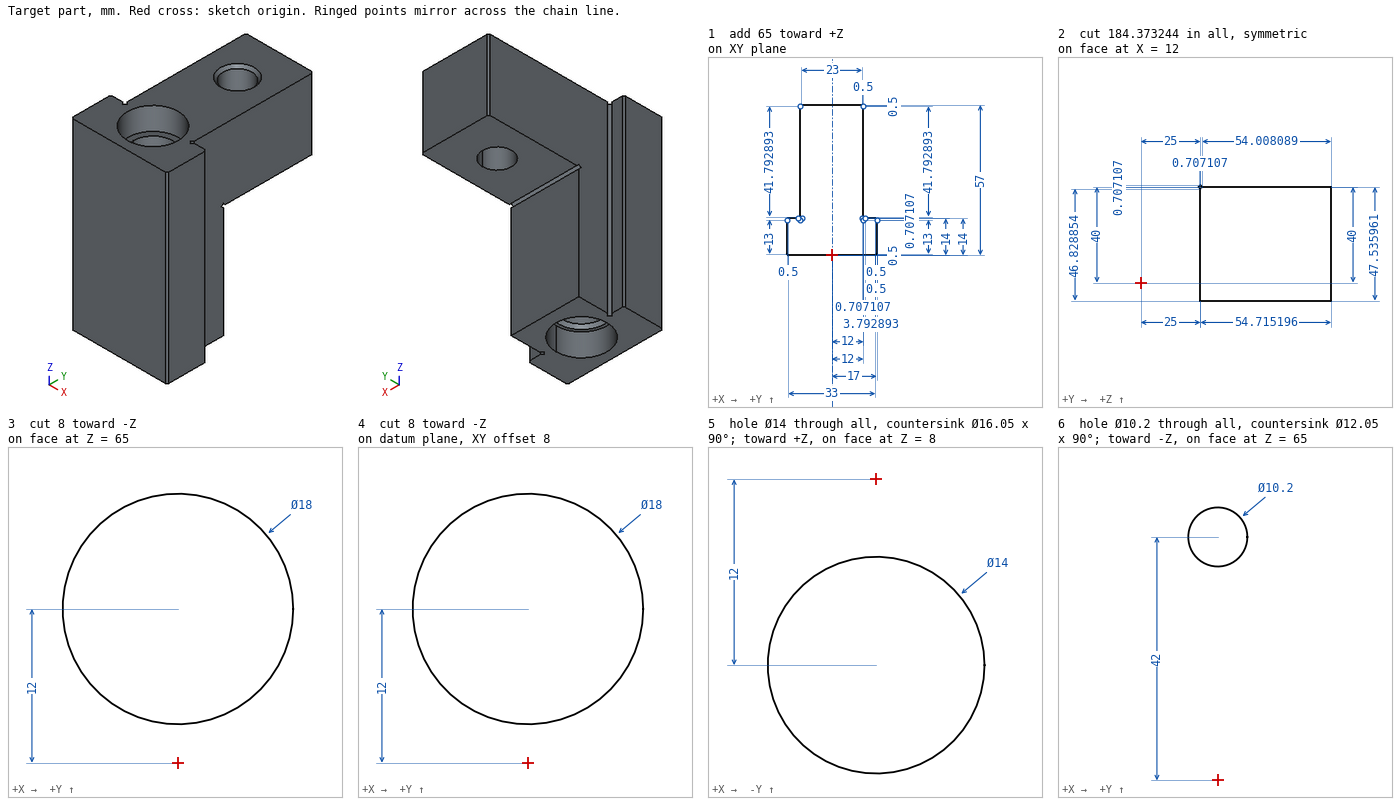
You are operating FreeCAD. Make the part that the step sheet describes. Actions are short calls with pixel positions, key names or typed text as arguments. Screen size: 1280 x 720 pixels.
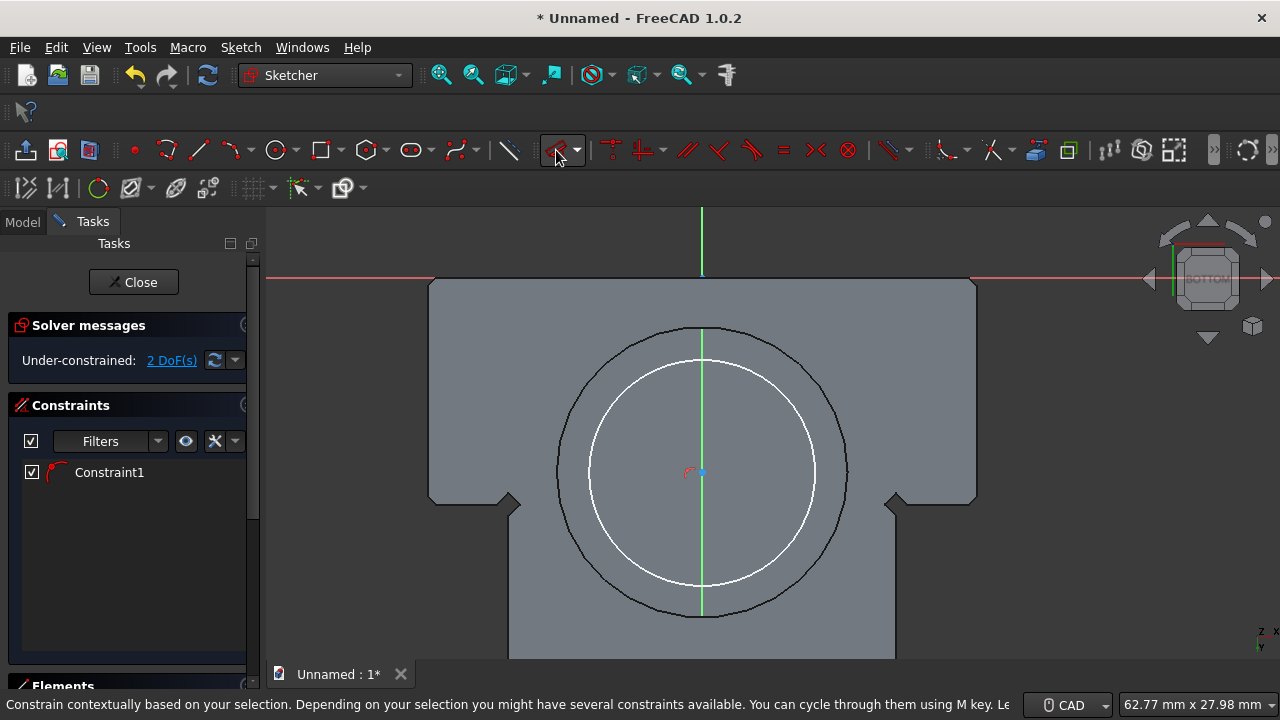
click(782, 393)
click(805, 370)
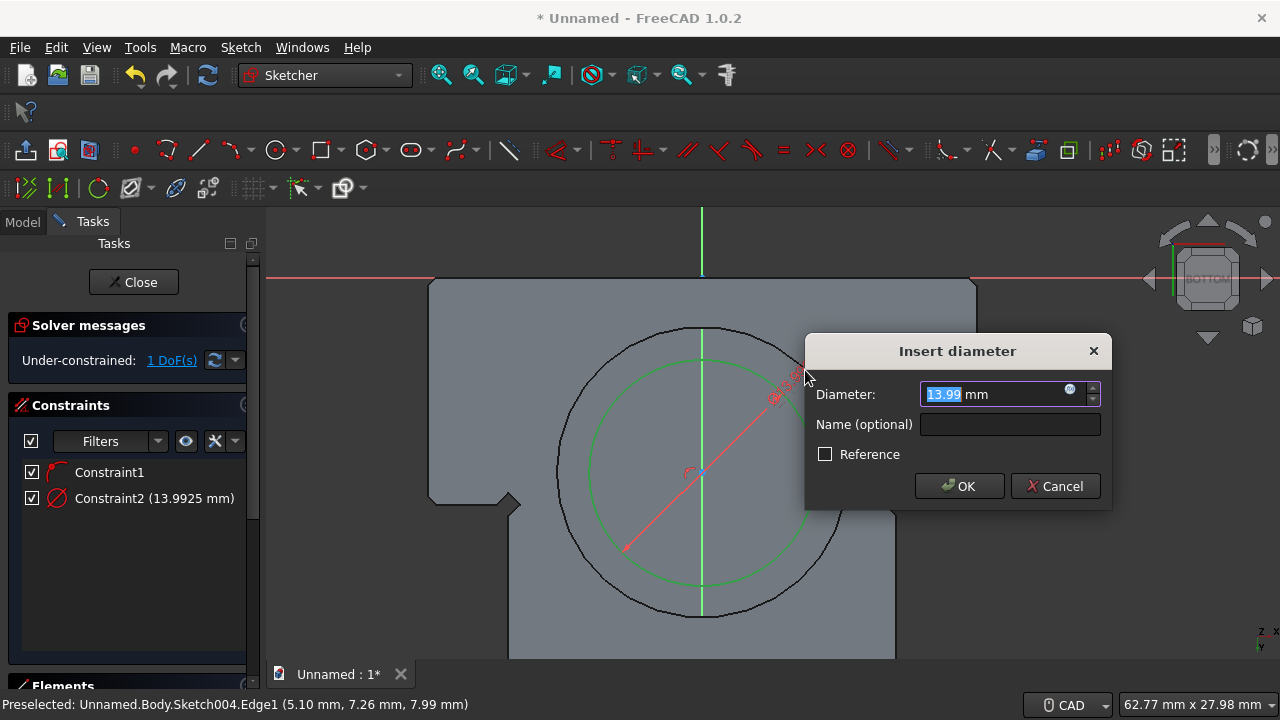
text(14)
key(Return)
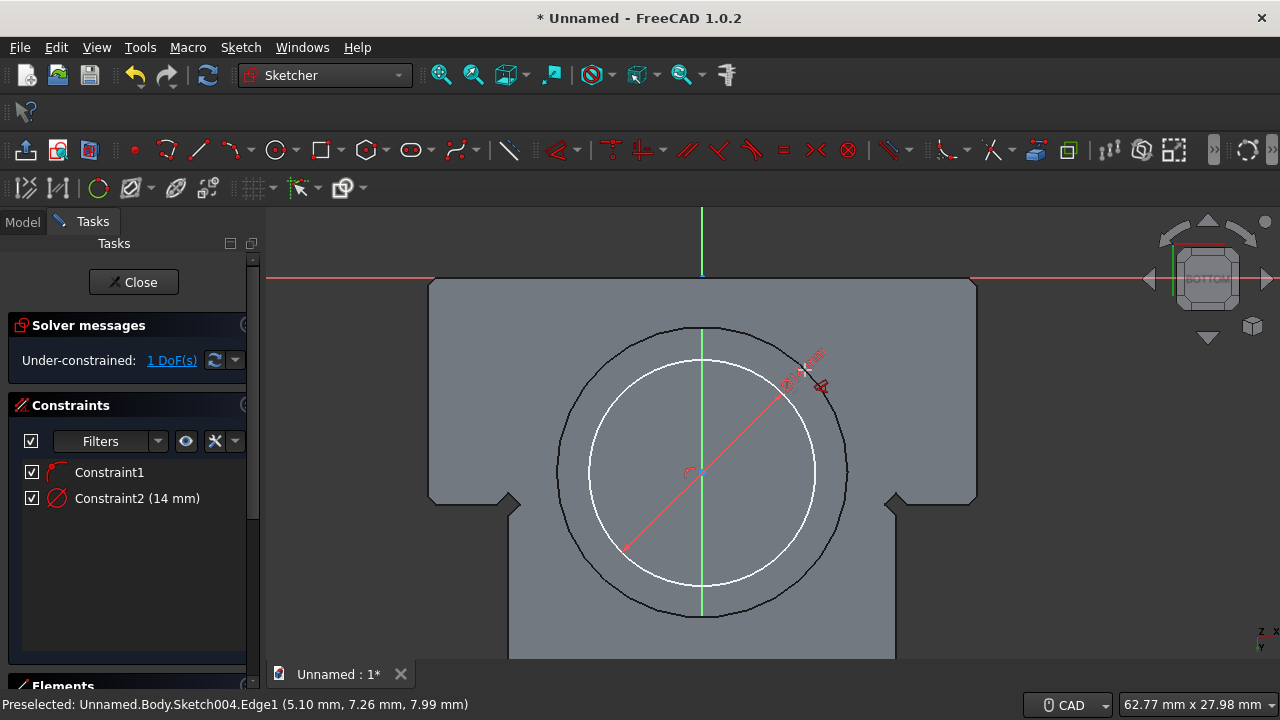
click(702, 473)
click(736, 331)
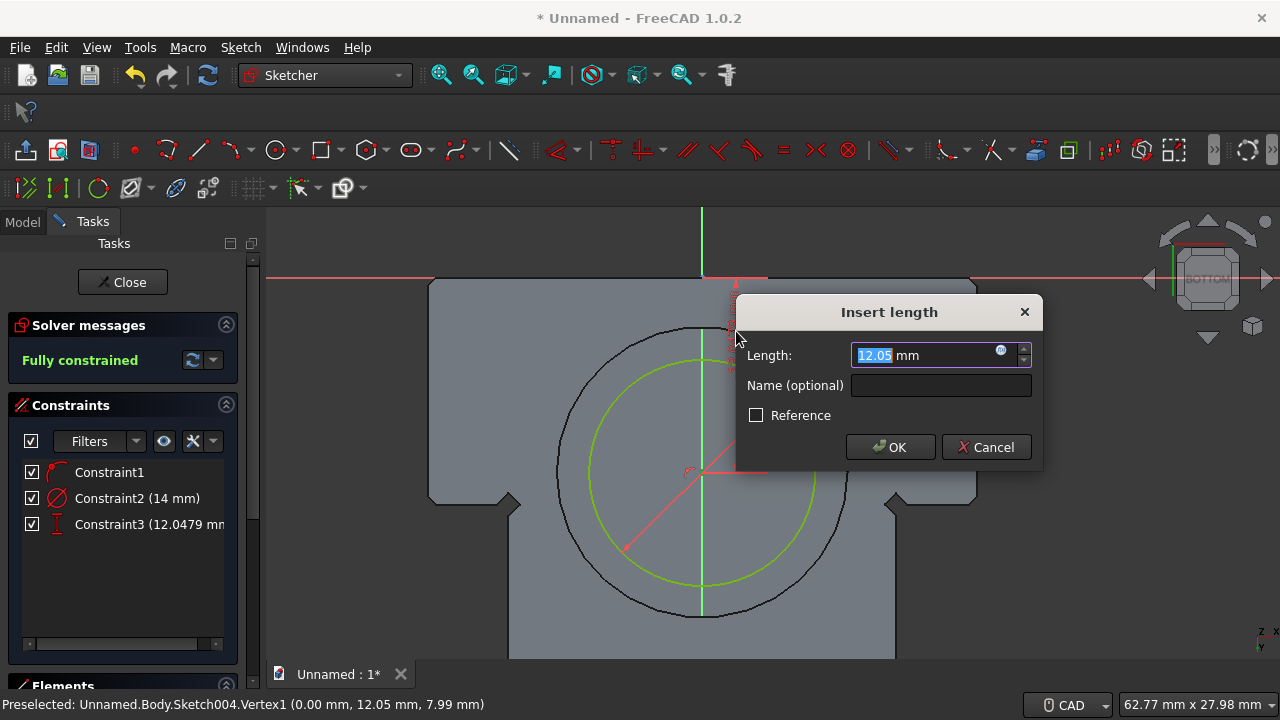
text(12)
key(Return)
key(Escape)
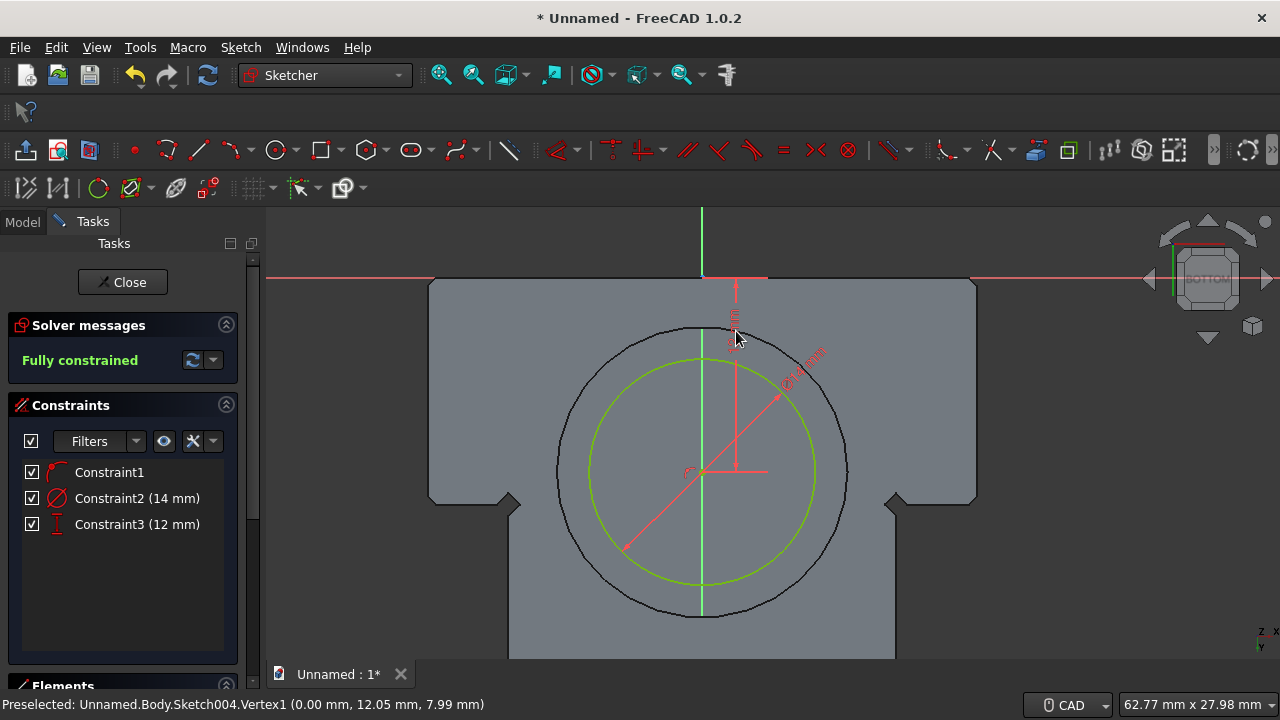
click(123, 282)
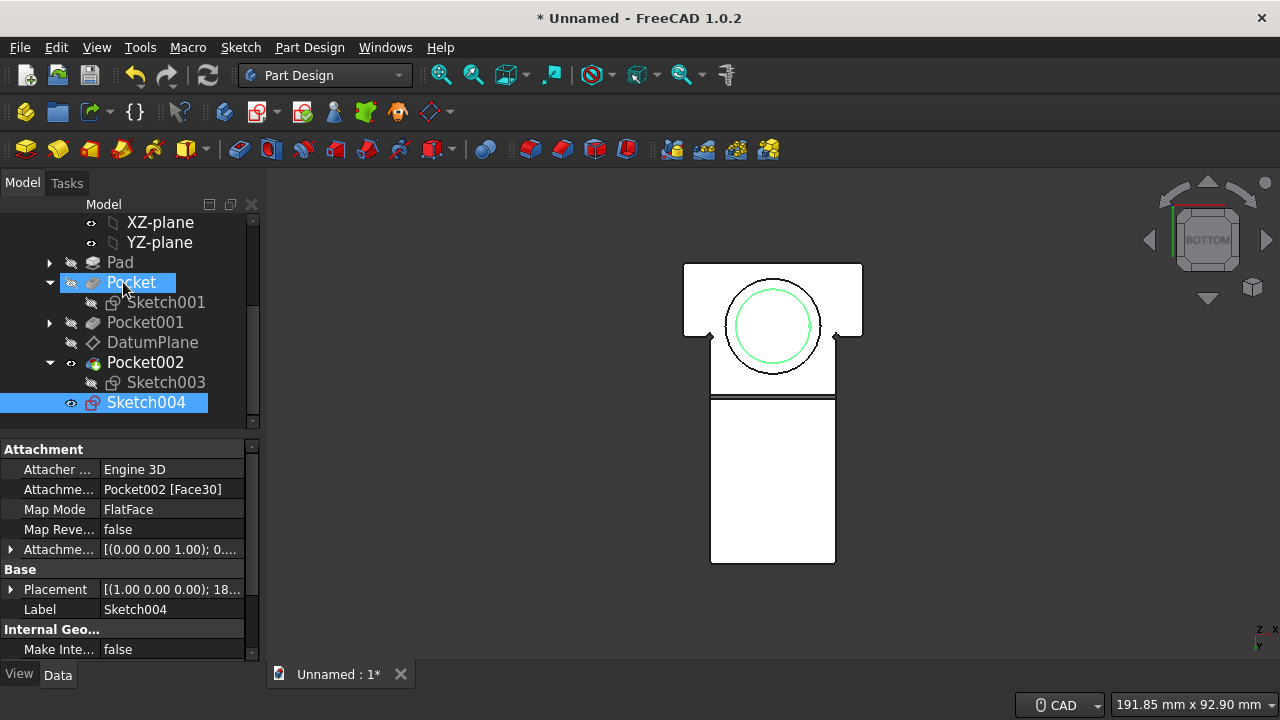
click(272, 150)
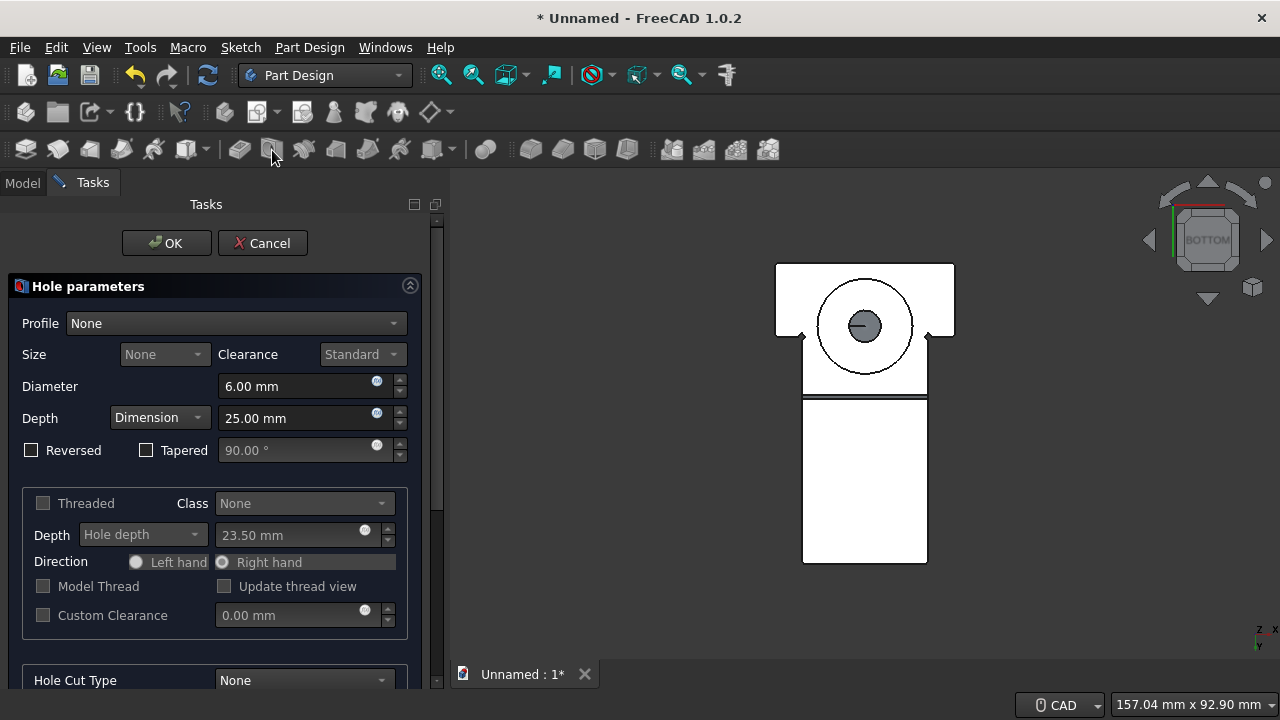
triple_click(305, 386)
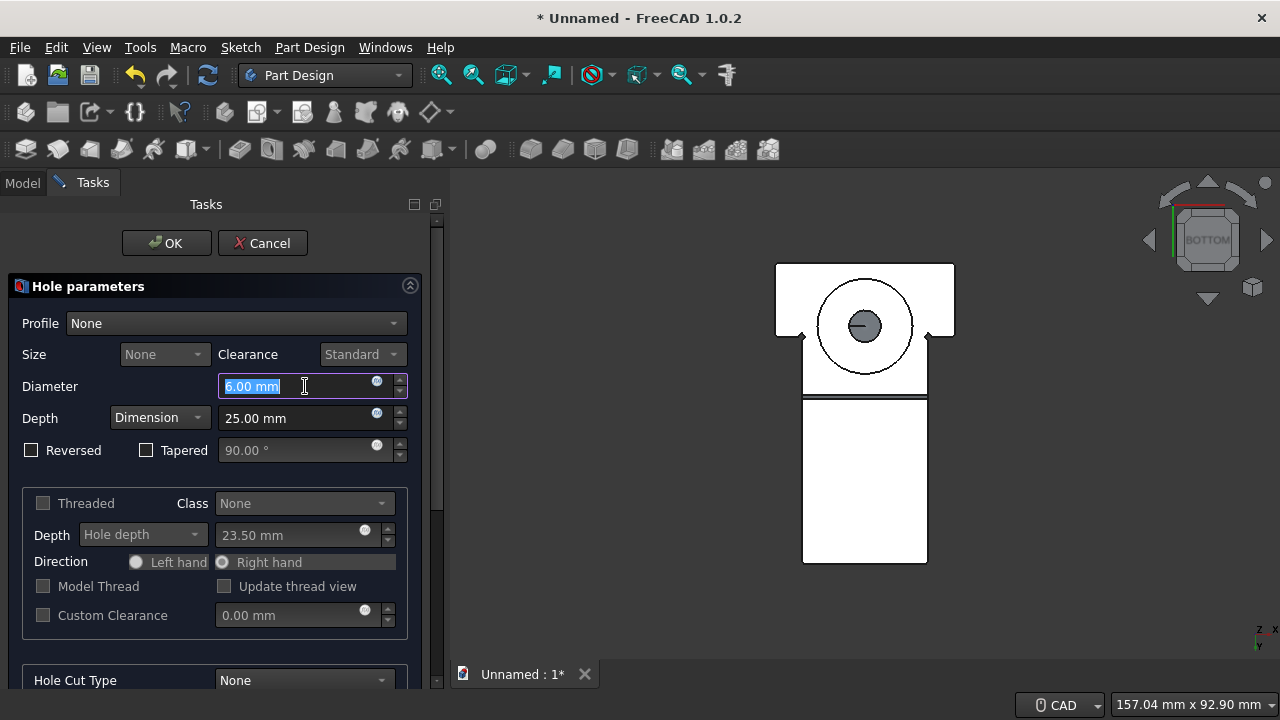
text(14)
key(Tab)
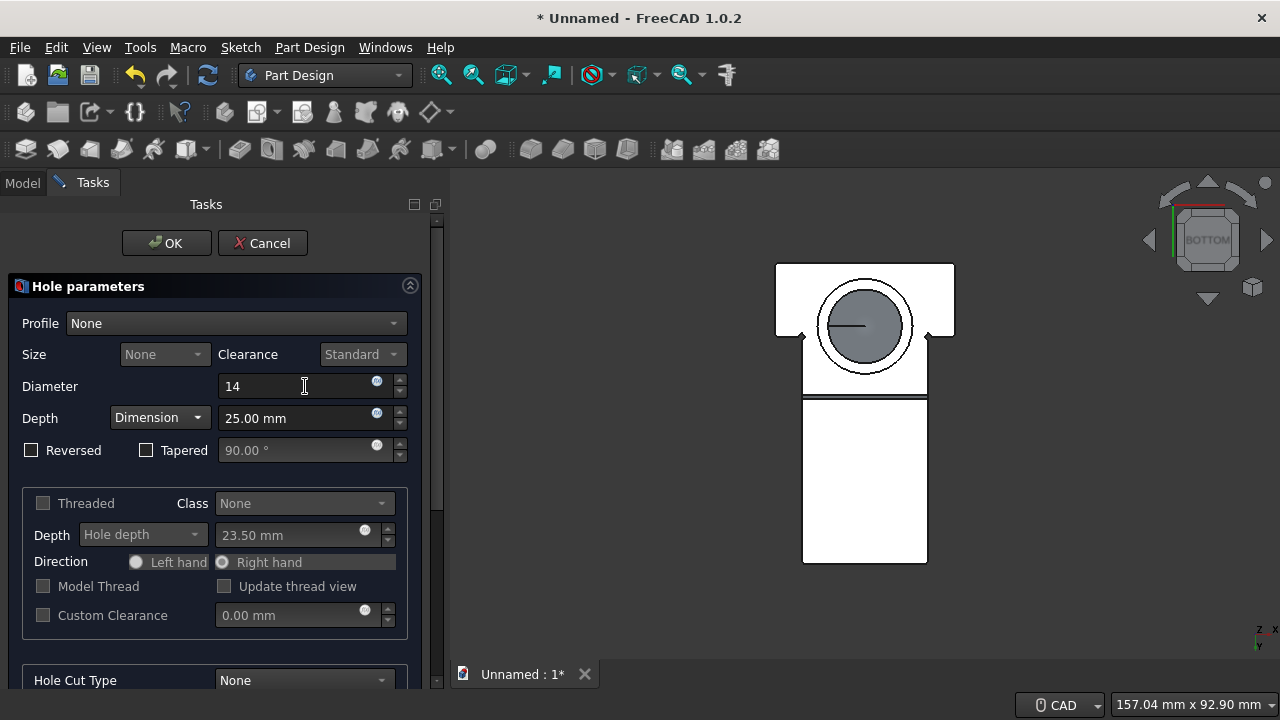
click(161, 418)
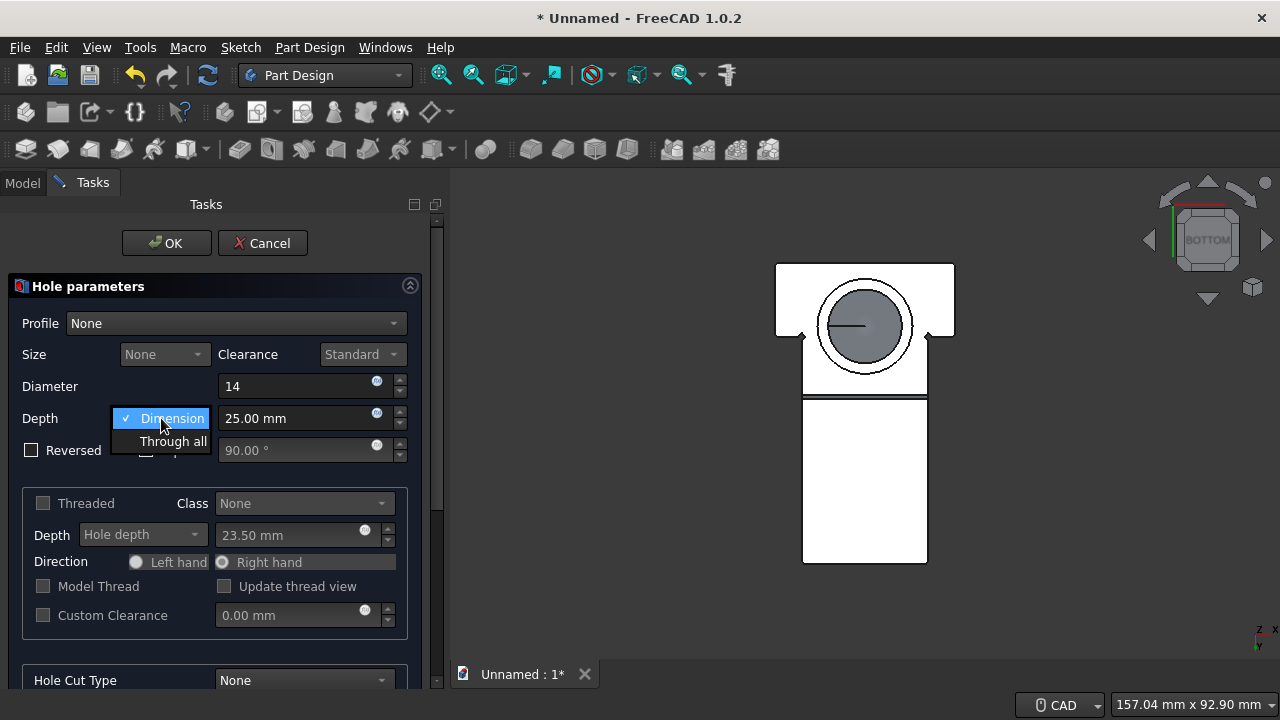
click(160, 442)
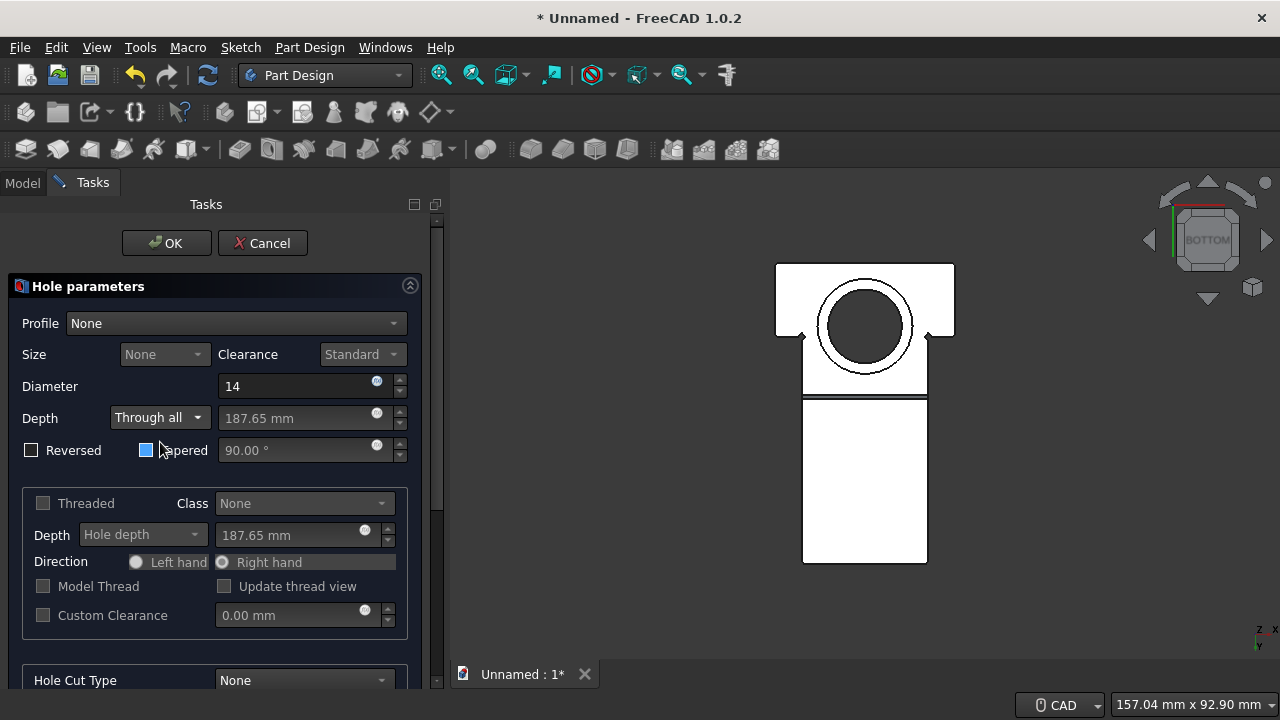
scroll(437, 451, down, 2)